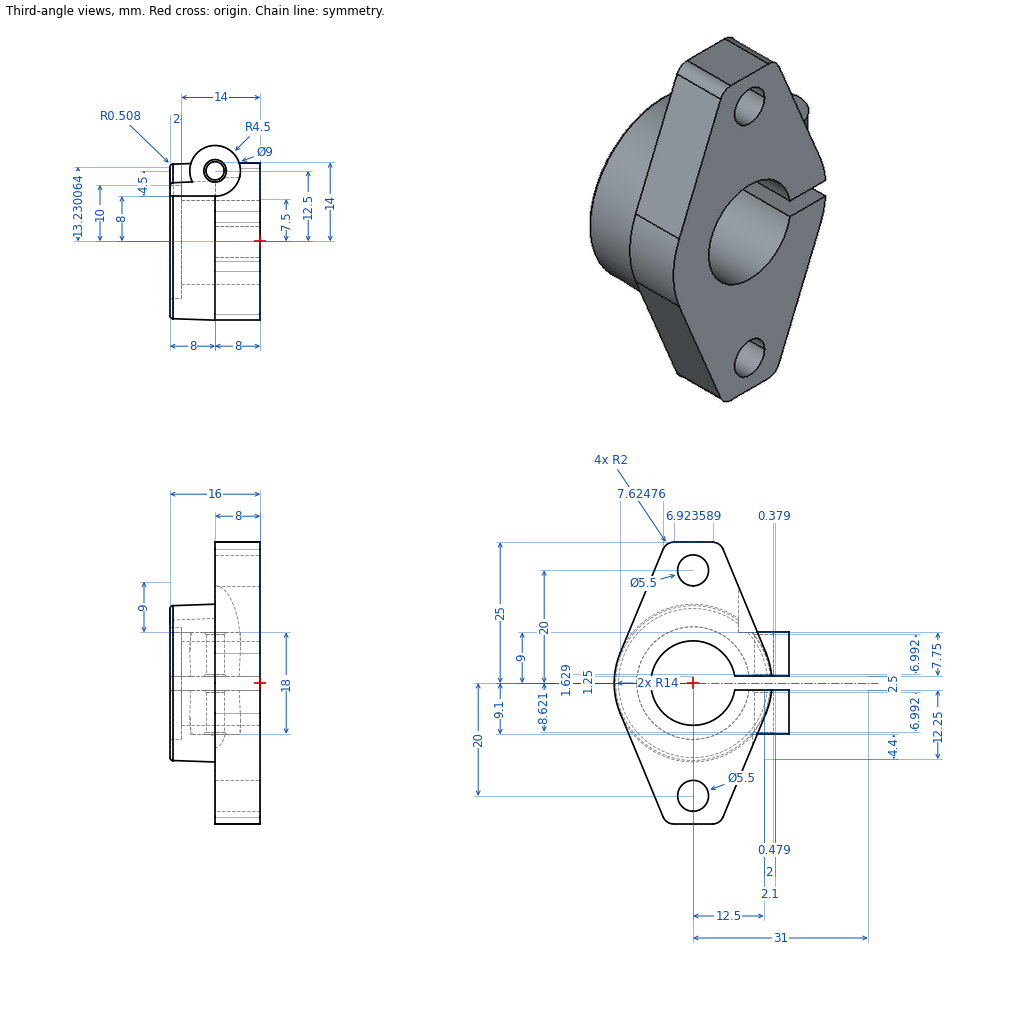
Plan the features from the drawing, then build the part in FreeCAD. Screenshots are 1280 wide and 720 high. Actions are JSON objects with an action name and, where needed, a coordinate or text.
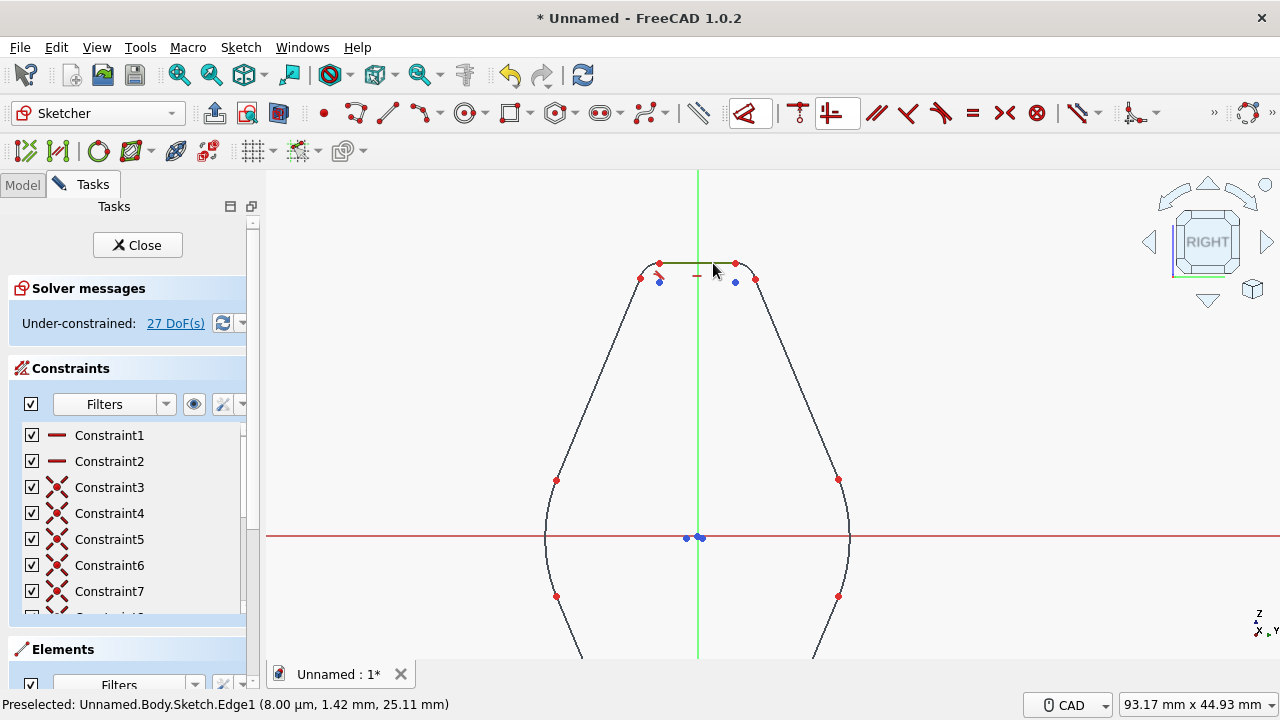
{"action": "left_click", "coordinate": [748, 268]}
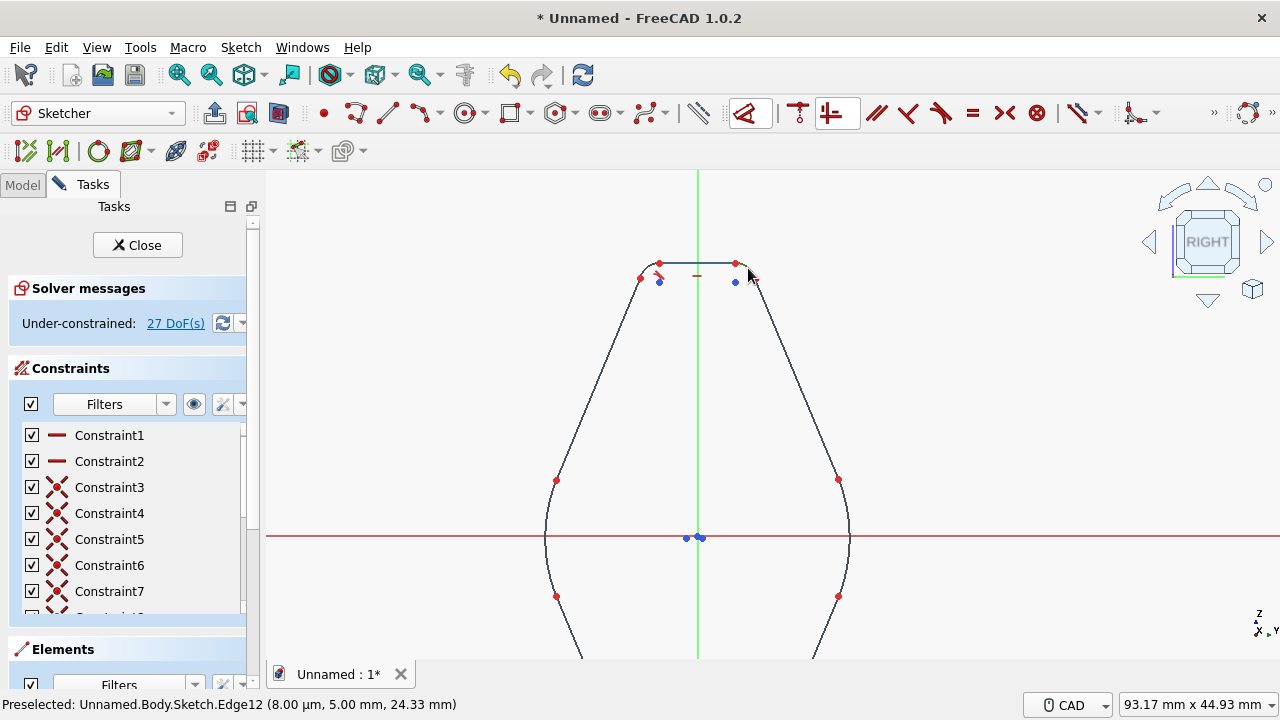
{"action": "left_click", "coordinate": [942, 114]}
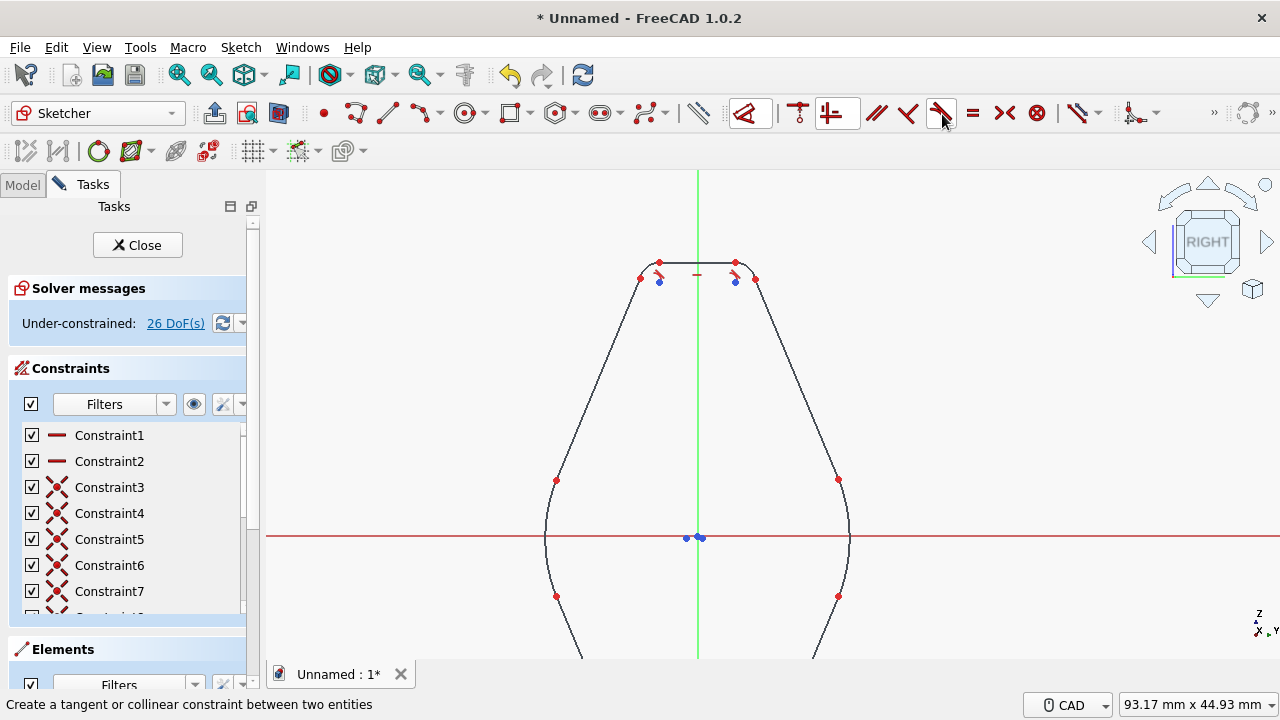
{"action": "left_click", "coordinate": [615, 339]}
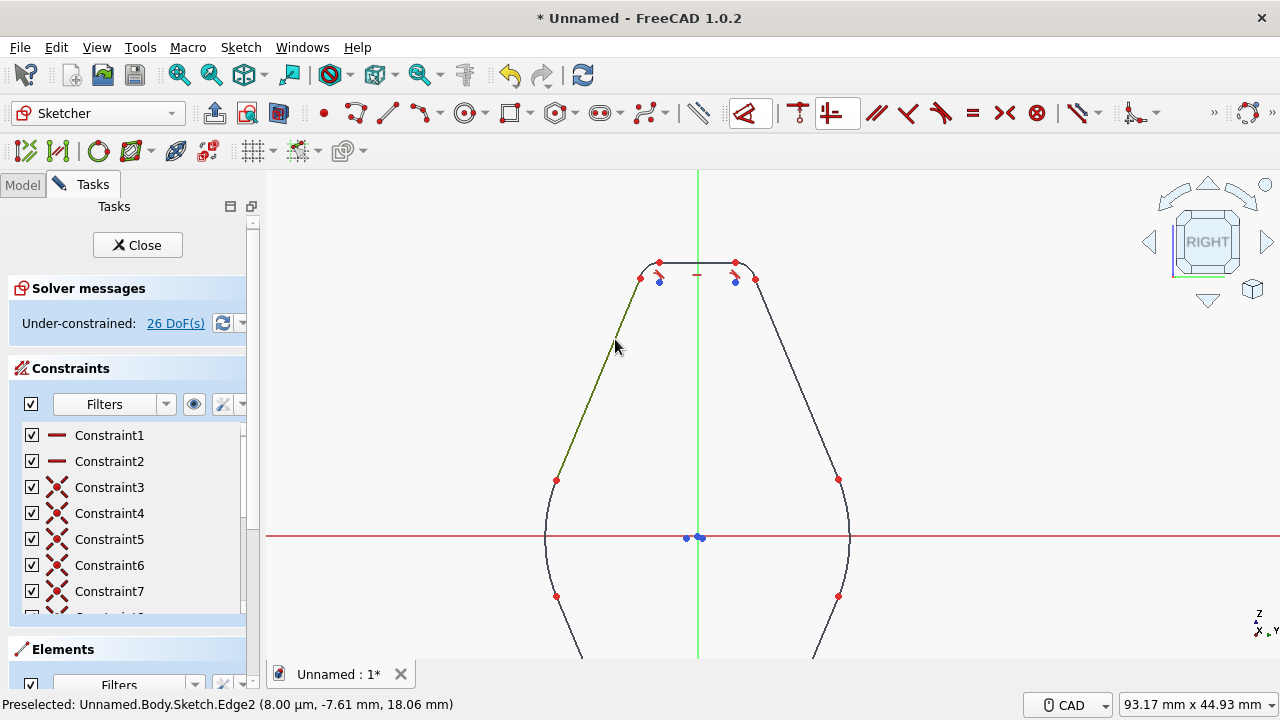
{"action": "left_click", "coordinate": [647, 267]}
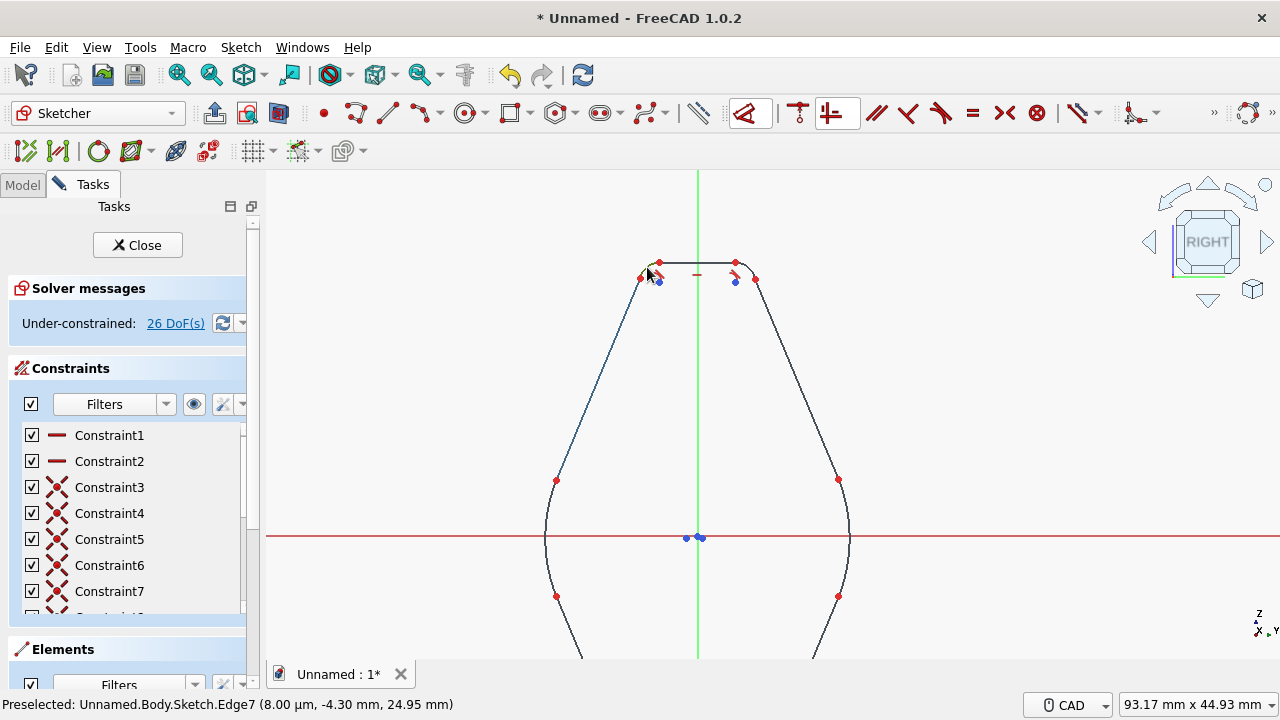
{"action": "left_click", "coordinate": [942, 114]}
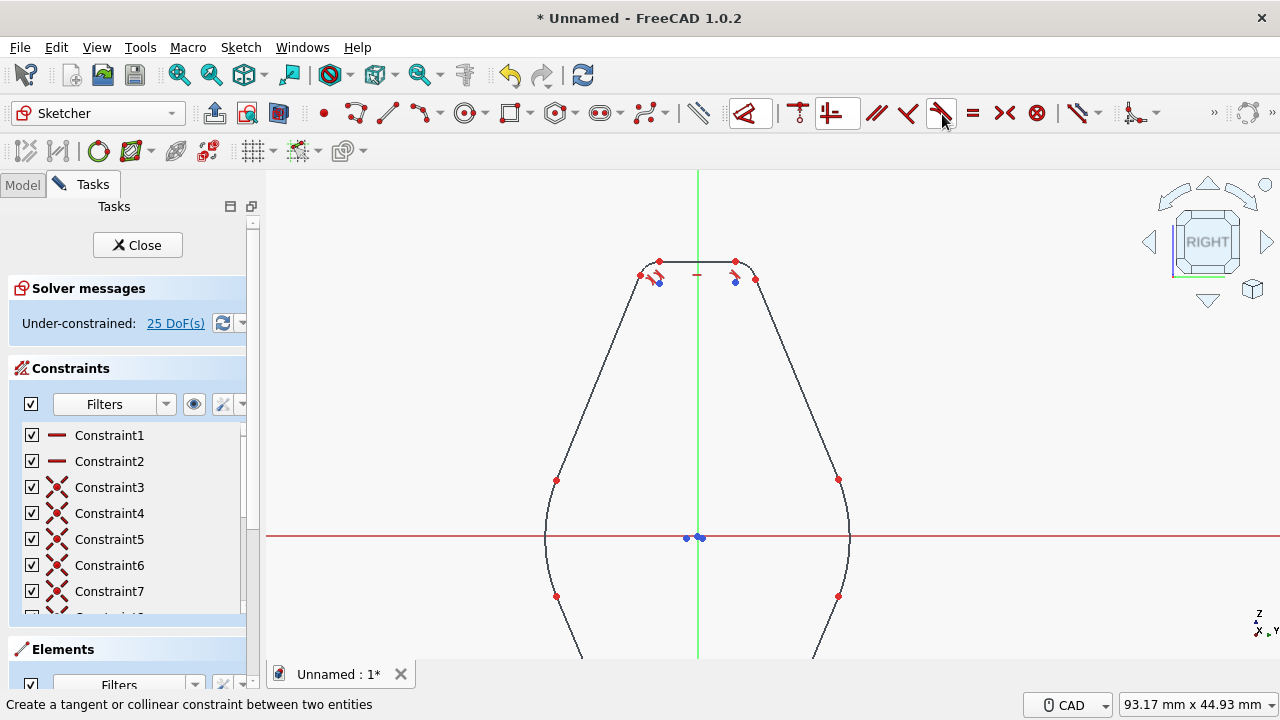
{"action": "left_click", "coordinate": [615, 337]}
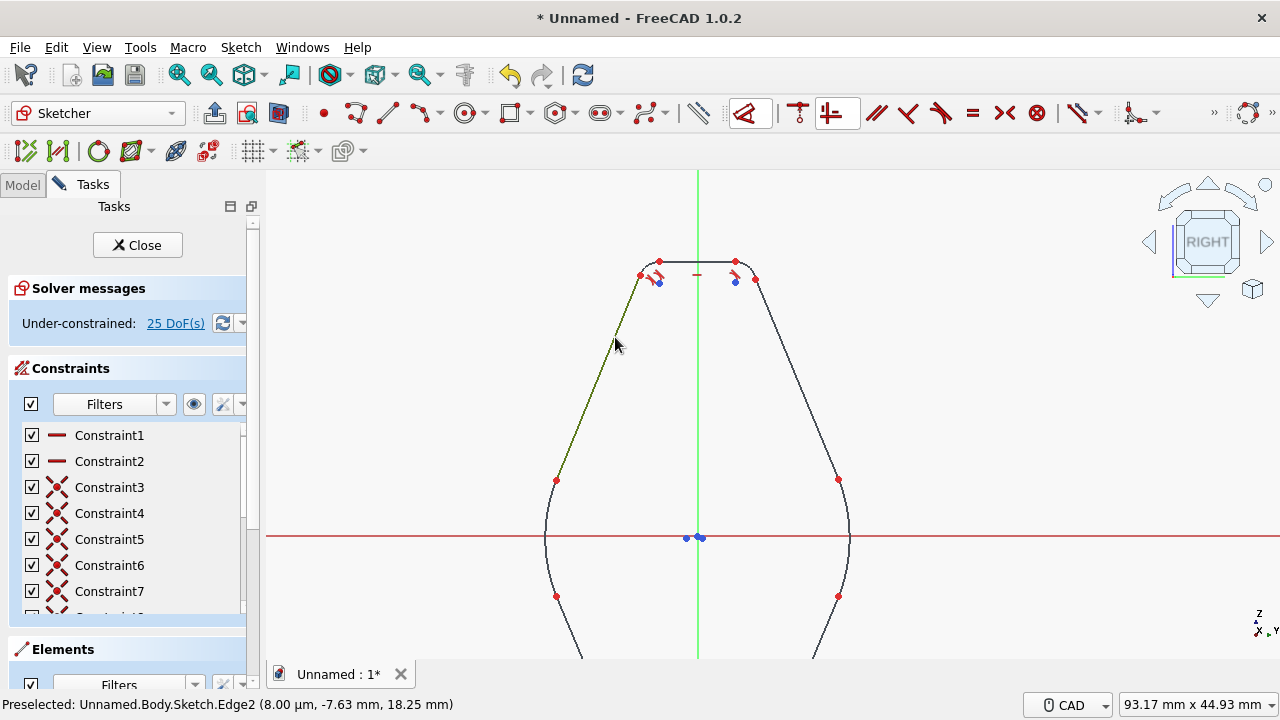
{"action": "left_click", "coordinate": [547, 515]}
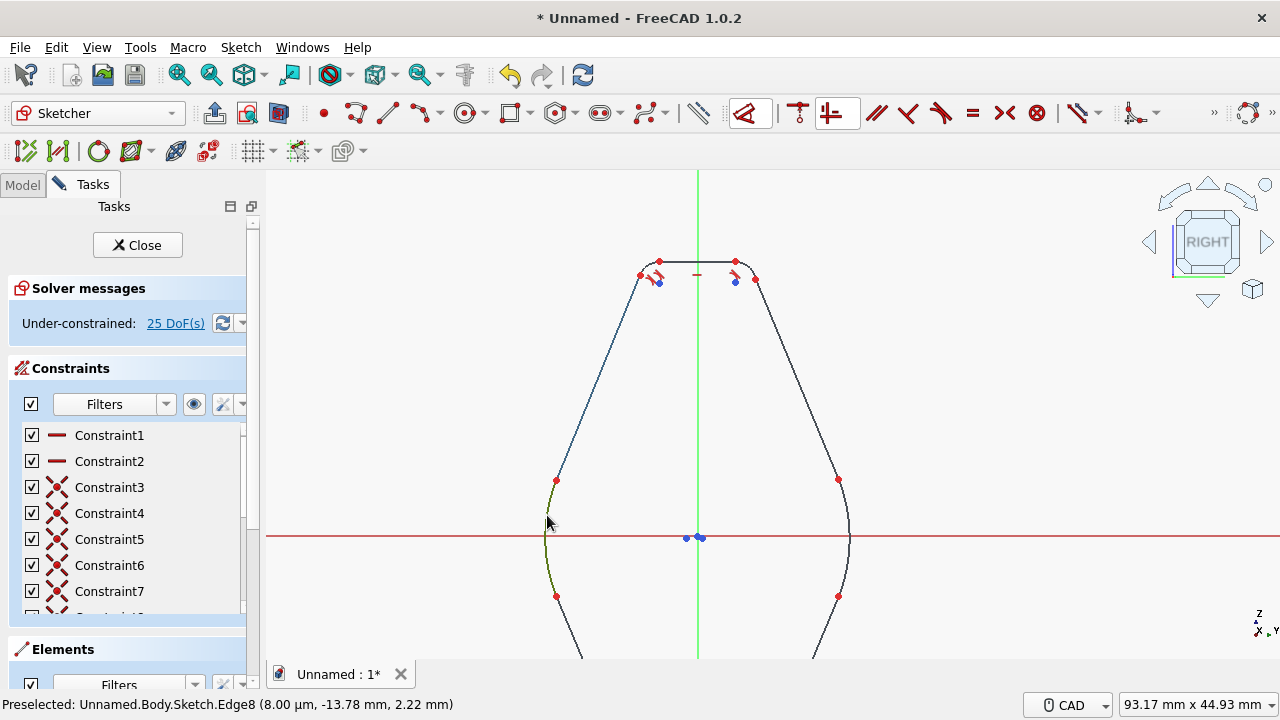
{"action": "left_click", "coordinate": [942, 114]}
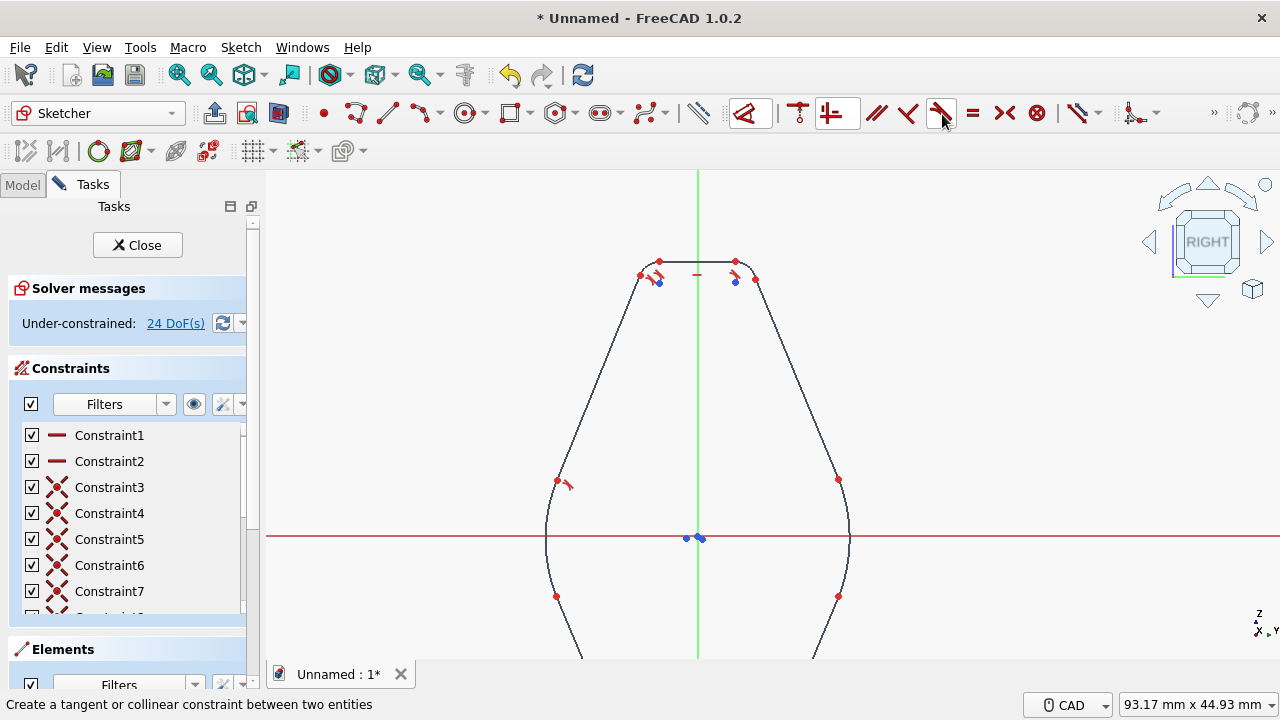
{"action": "scroll", "coordinate": [713, 266], "scroll_direction": "down", "scroll_amount": 3}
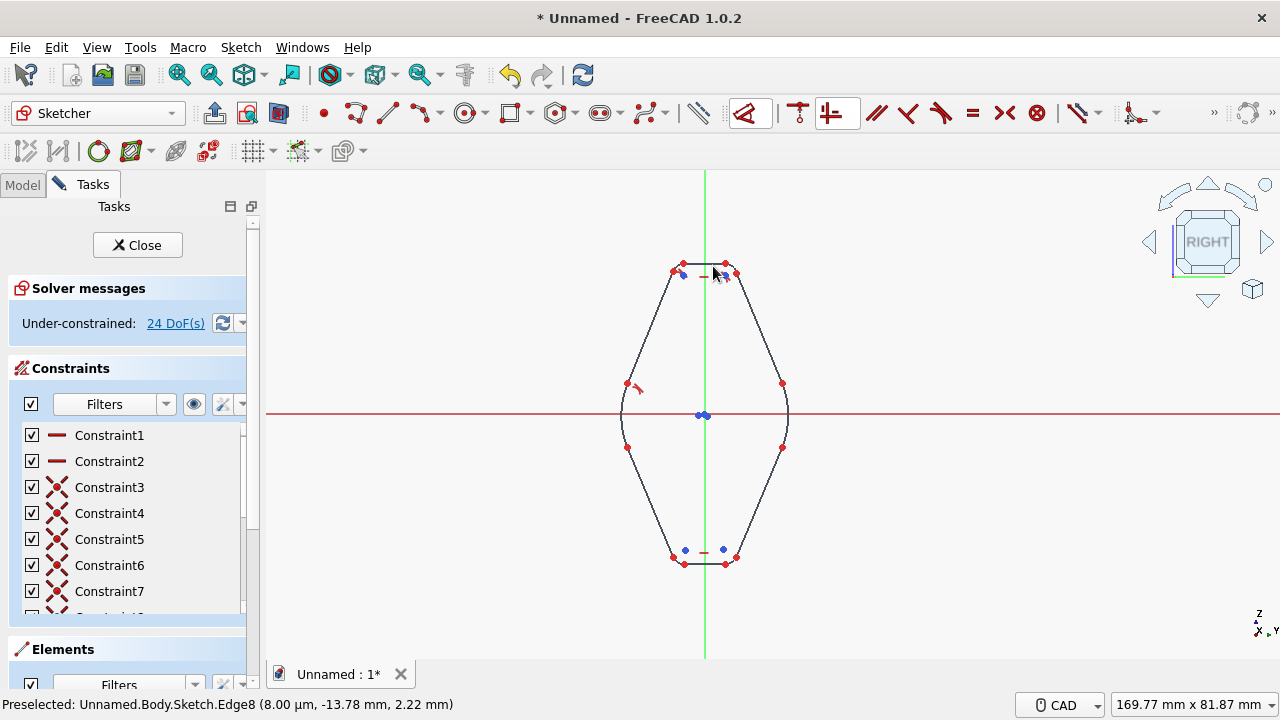
{"action": "left_click", "coordinate": [641, 480]}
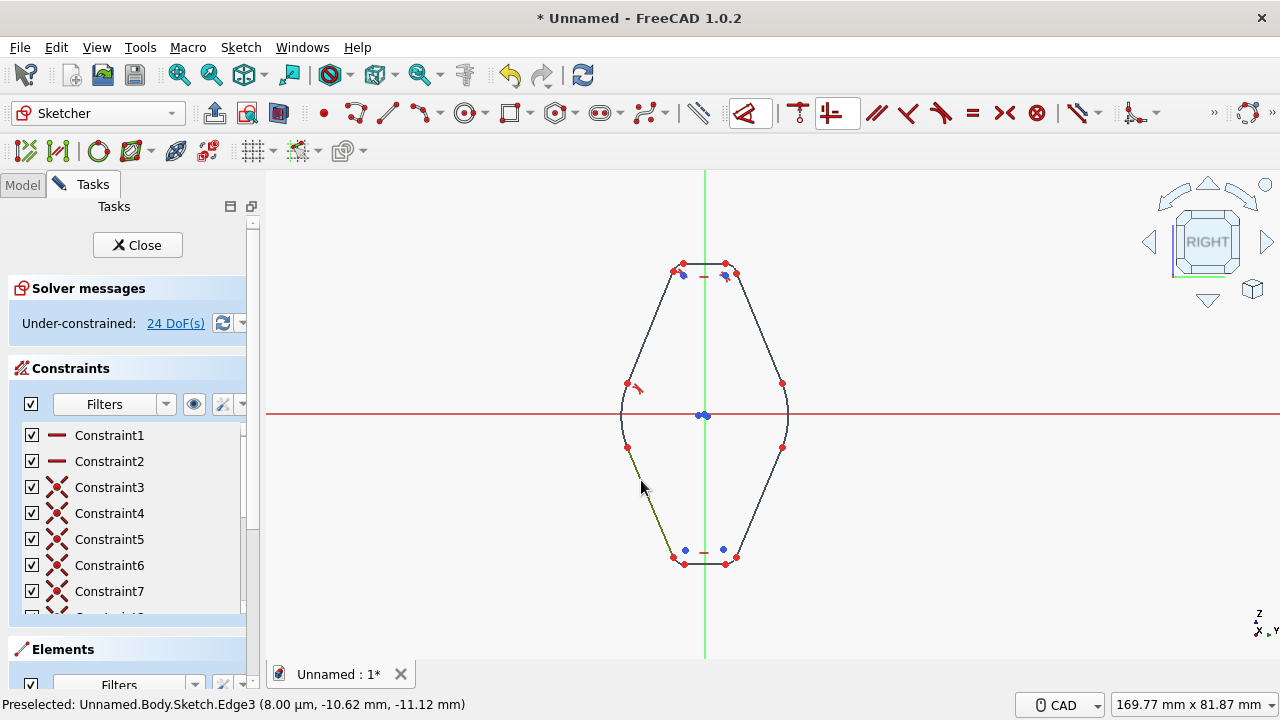
{"action": "left_click", "coordinate": [622, 403]}